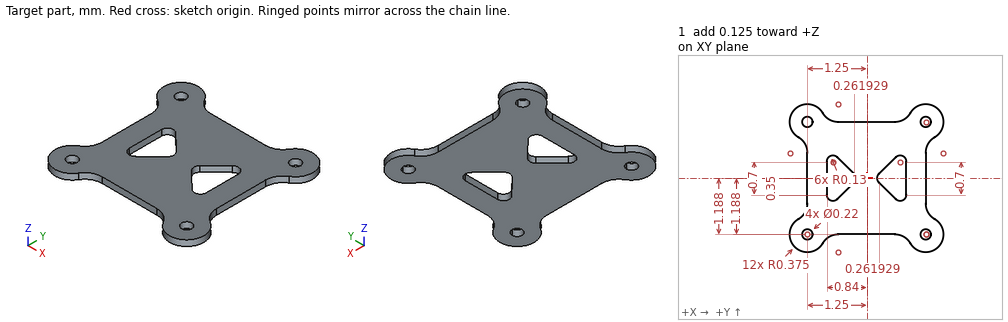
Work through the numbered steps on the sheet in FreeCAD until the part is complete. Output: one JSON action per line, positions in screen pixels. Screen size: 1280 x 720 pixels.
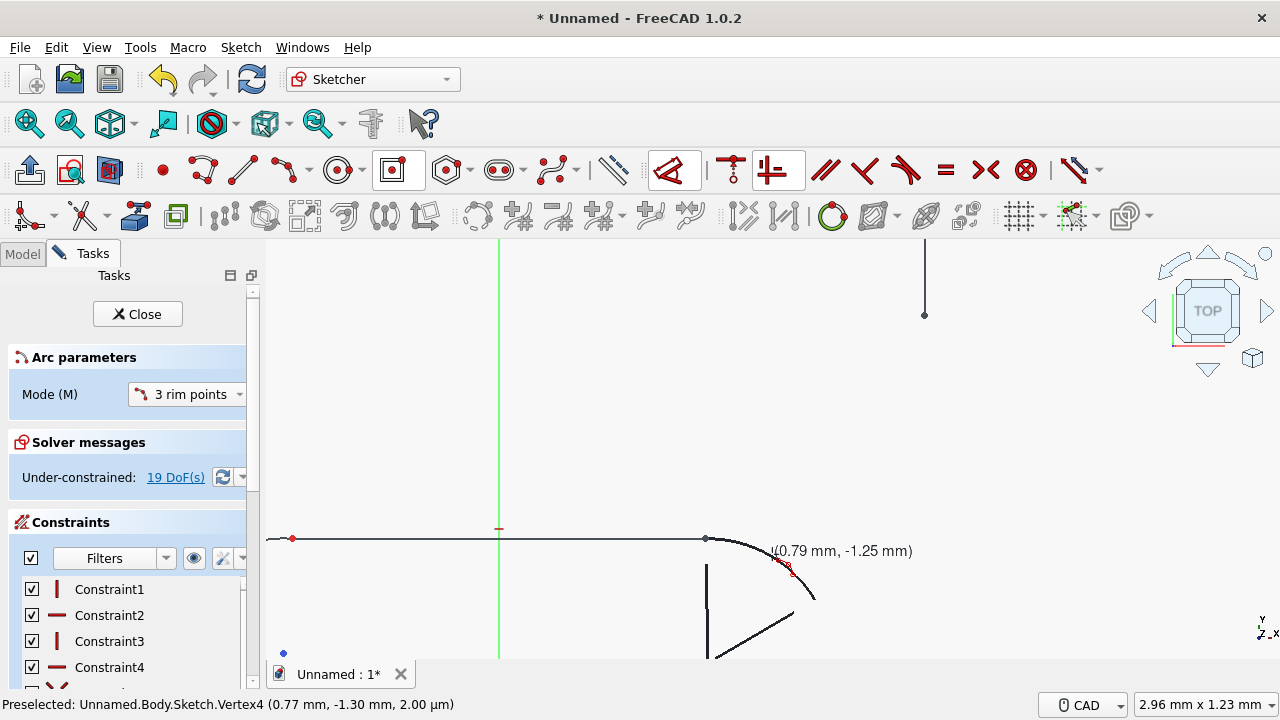
{"action": "left_click", "coordinate": [769, 551]}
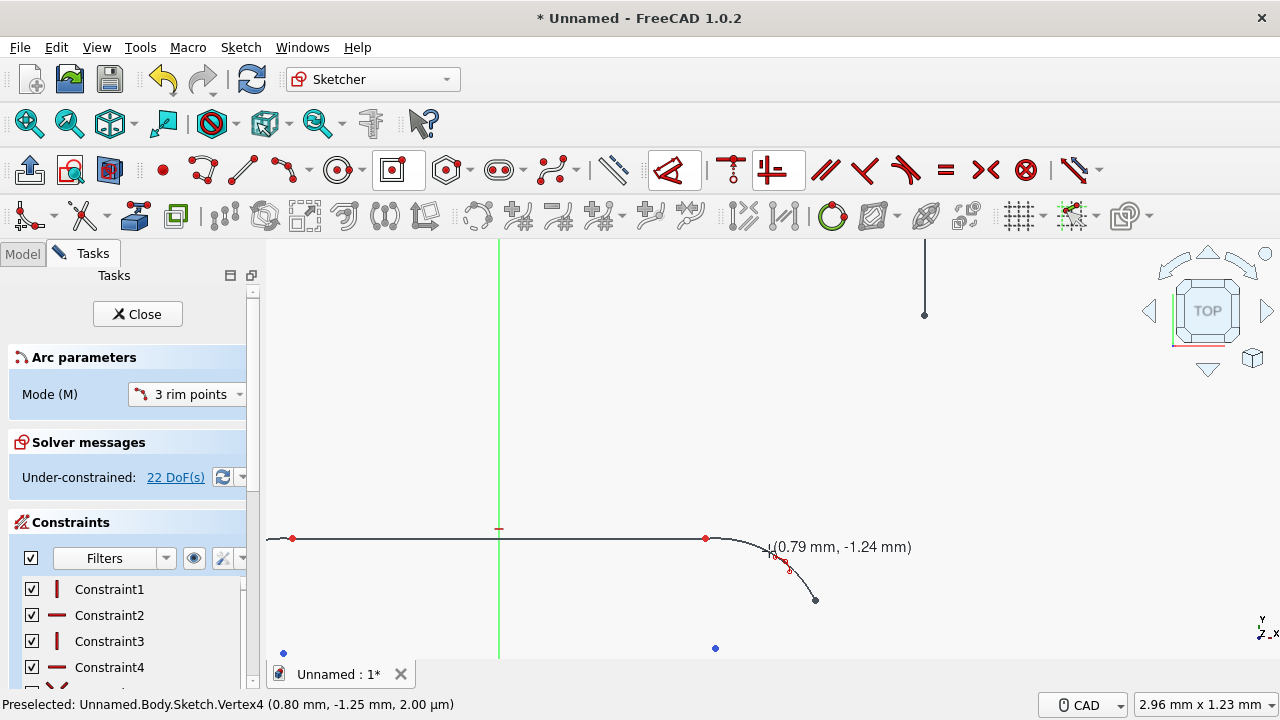
{"action": "scroll", "coordinate": [772, 554], "scroll_direction": "down", "scroll_amount": 7}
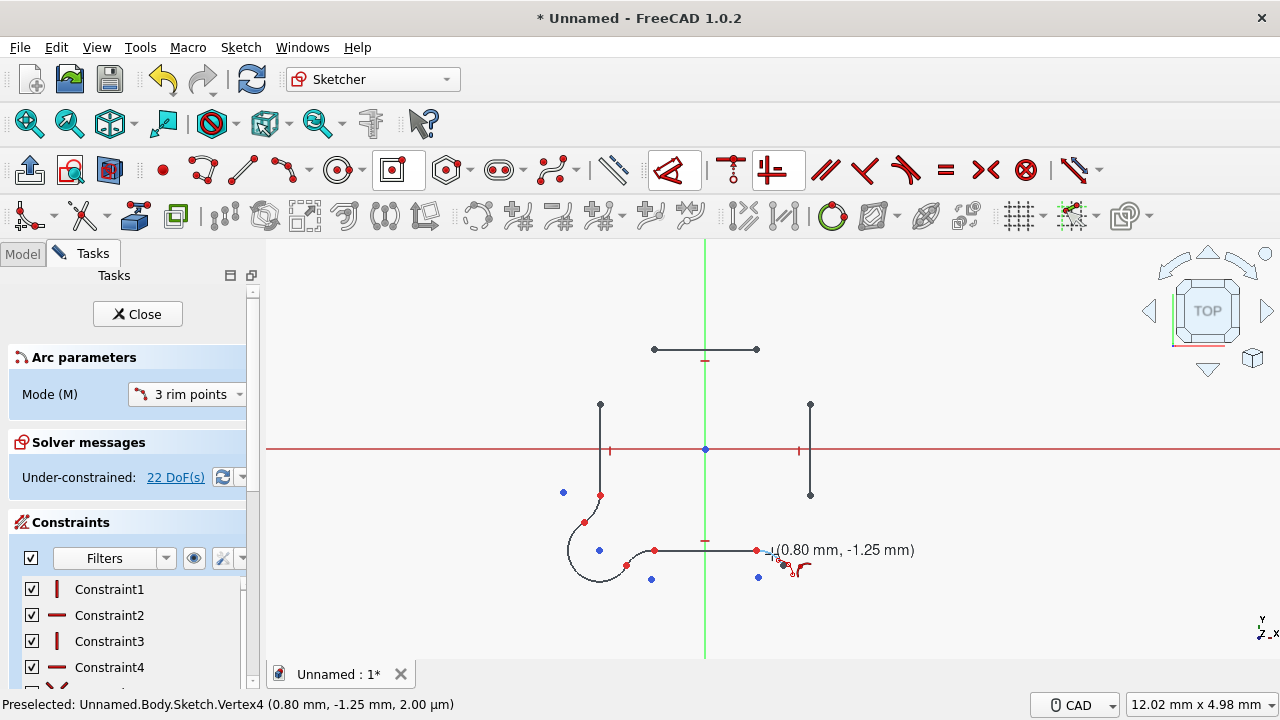
{"action": "left_click", "coordinate": [783, 566]}
{"action": "left_click", "coordinate": [826, 522]}
{"action": "left_click", "coordinate": [833, 572]}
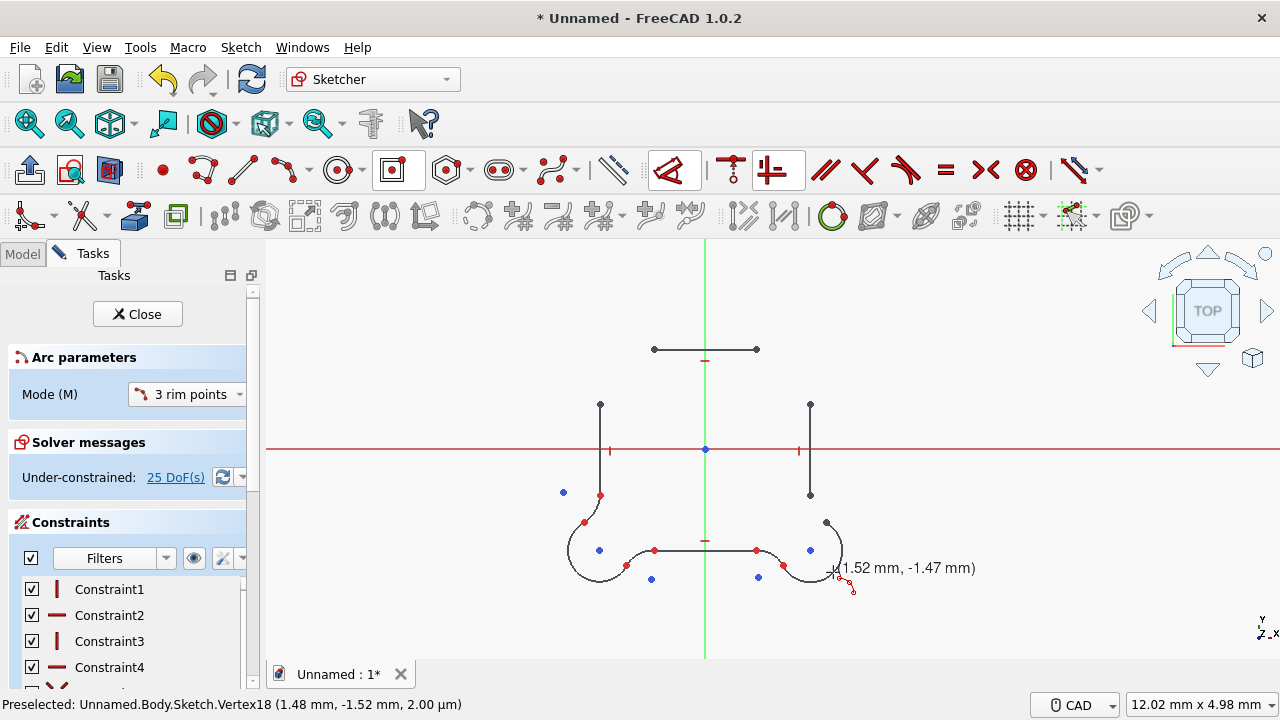
{"action": "left_click", "coordinate": [826, 523]}
{"action": "left_click", "coordinate": [810, 496]}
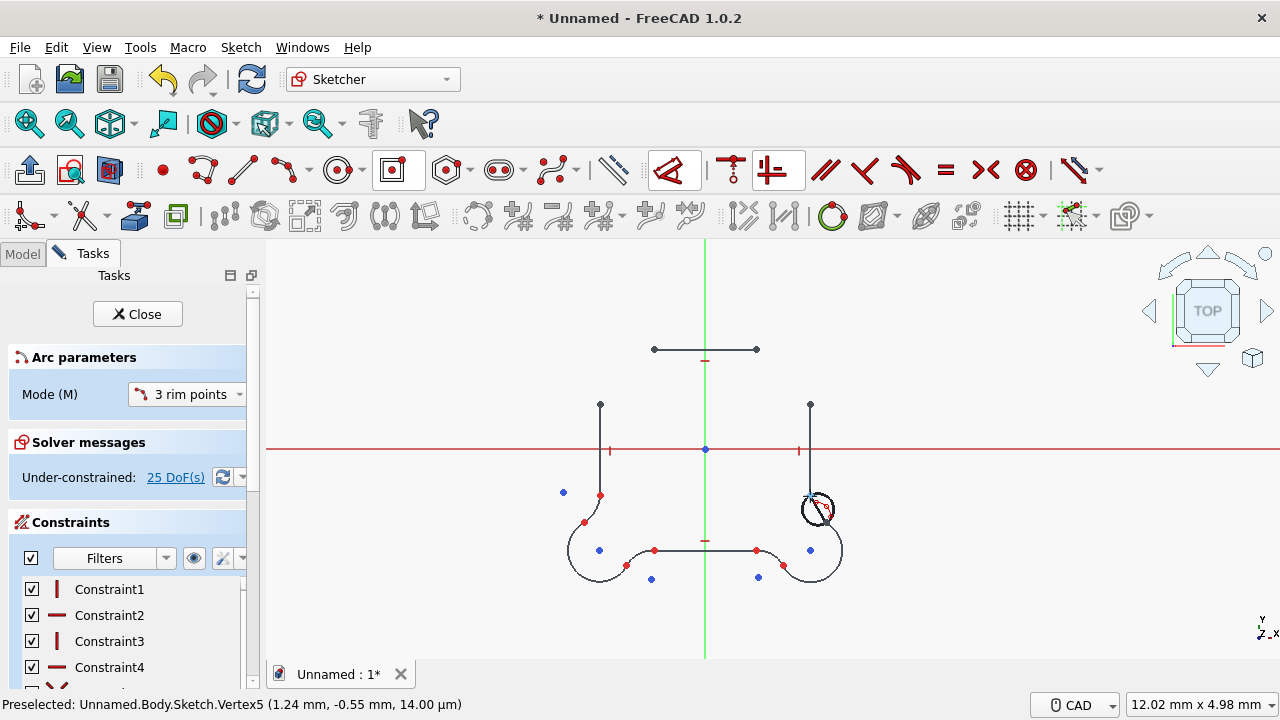
{"action": "scroll", "coordinate": [815, 510], "scroll_direction": "up", "scroll_amount": 7}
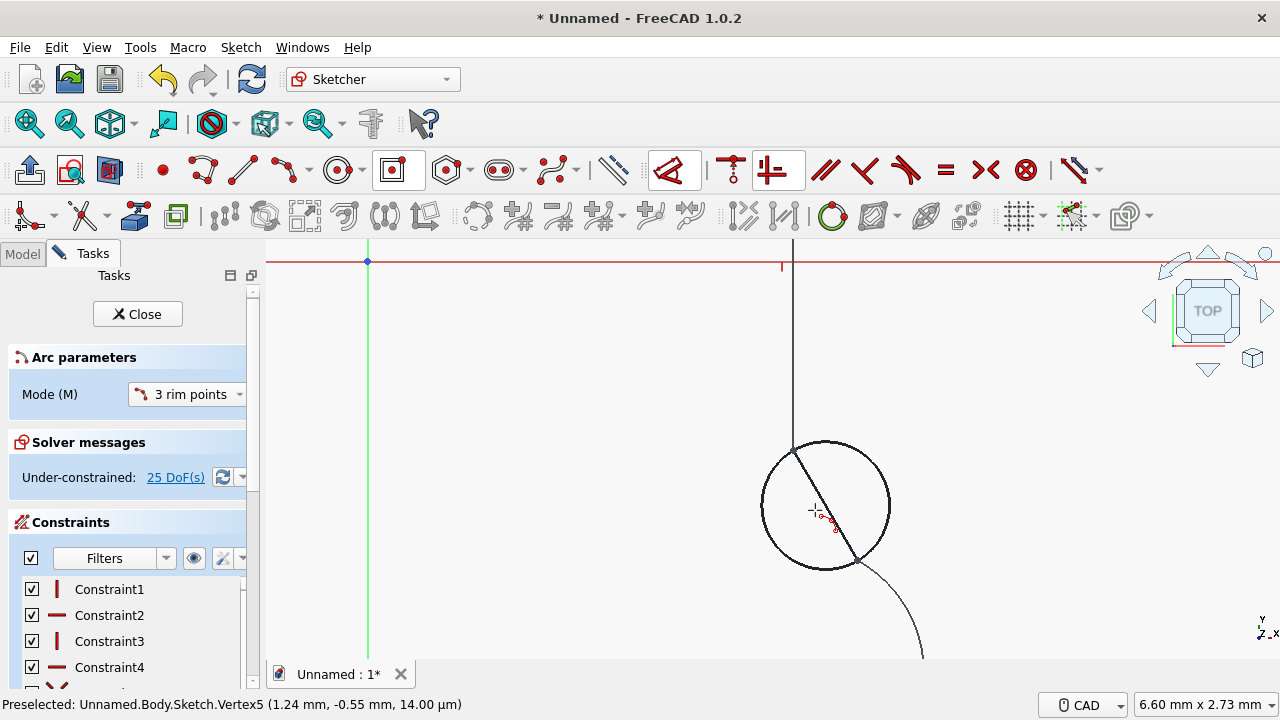
{"action": "left_click", "coordinate": [813, 510]}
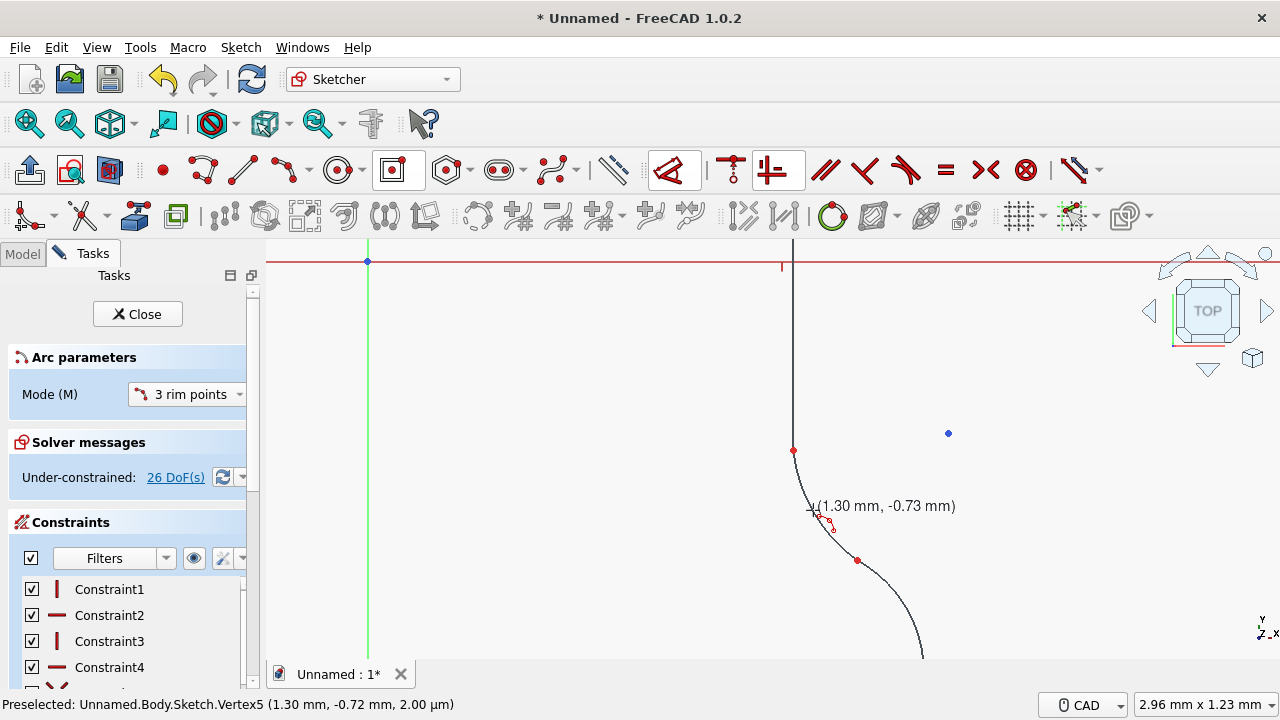
{"action": "scroll", "coordinate": [815, 510], "scroll_direction": "down", "scroll_amount": 7}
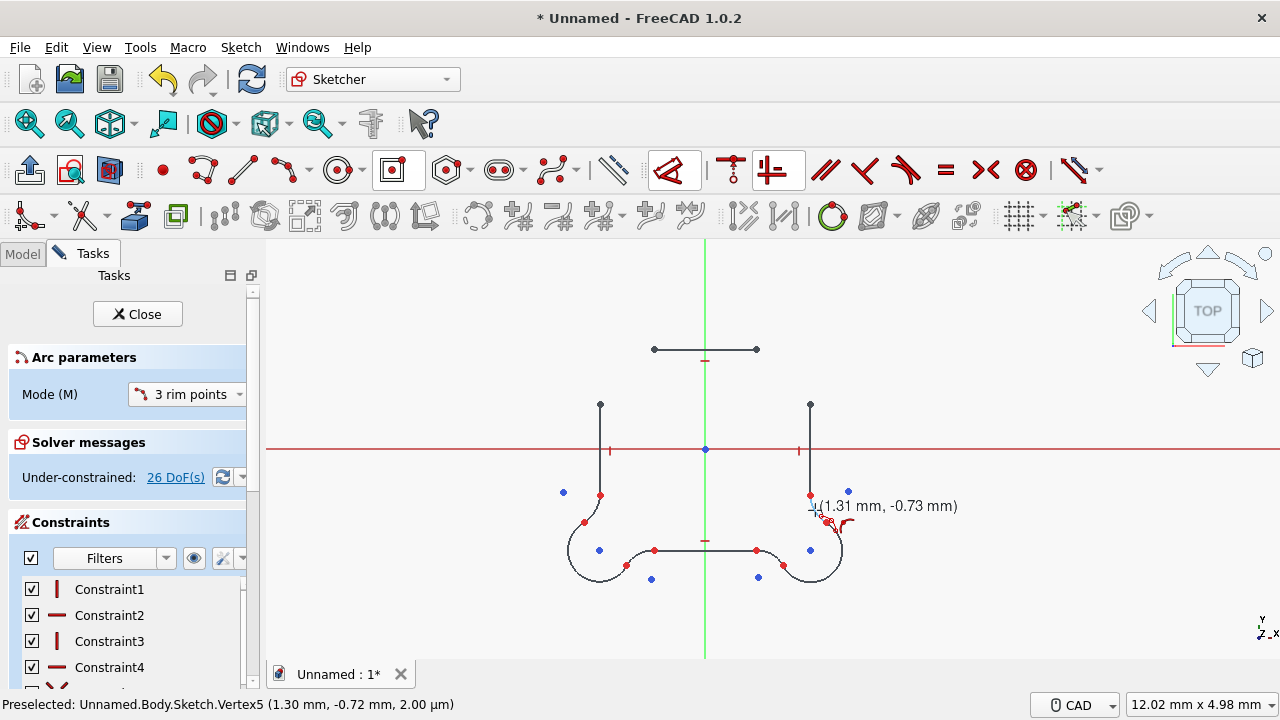
{"action": "left_click", "coordinate": [810, 405]}
{"action": "left_click", "coordinate": [826, 376]}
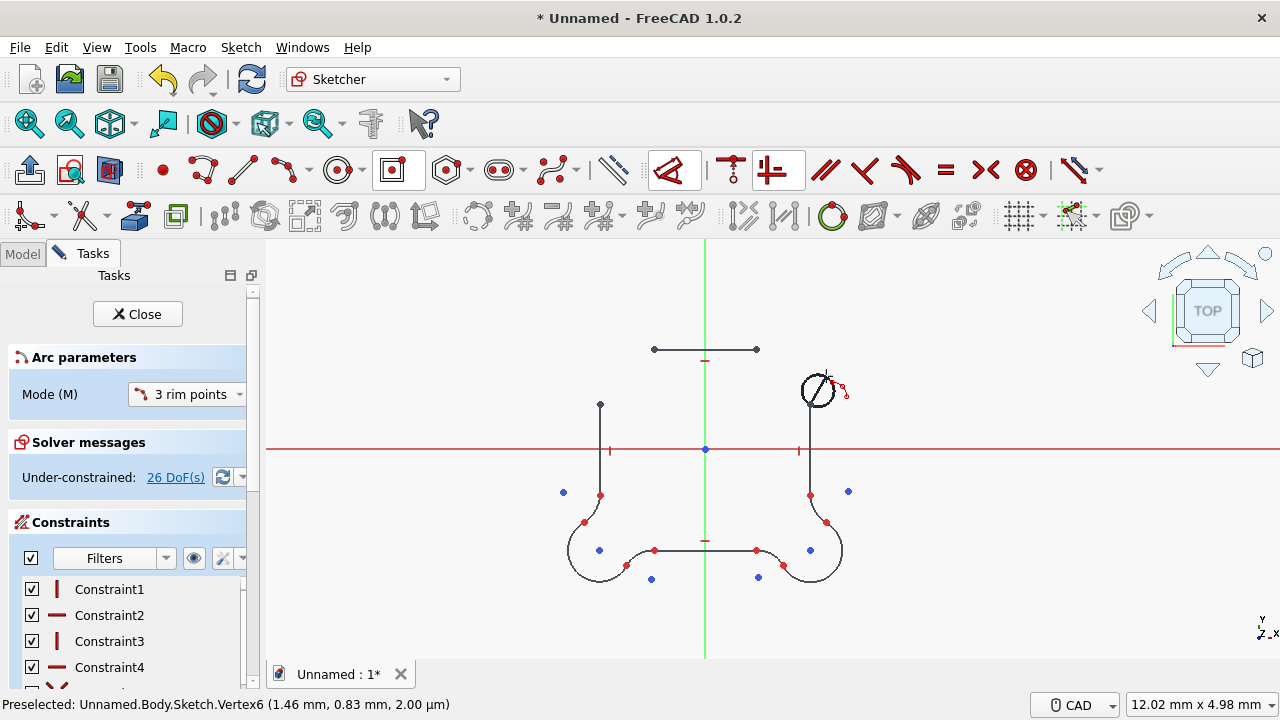
{"action": "scroll", "coordinate": [815, 388], "scroll_direction": "up", "scroll_amount": 7}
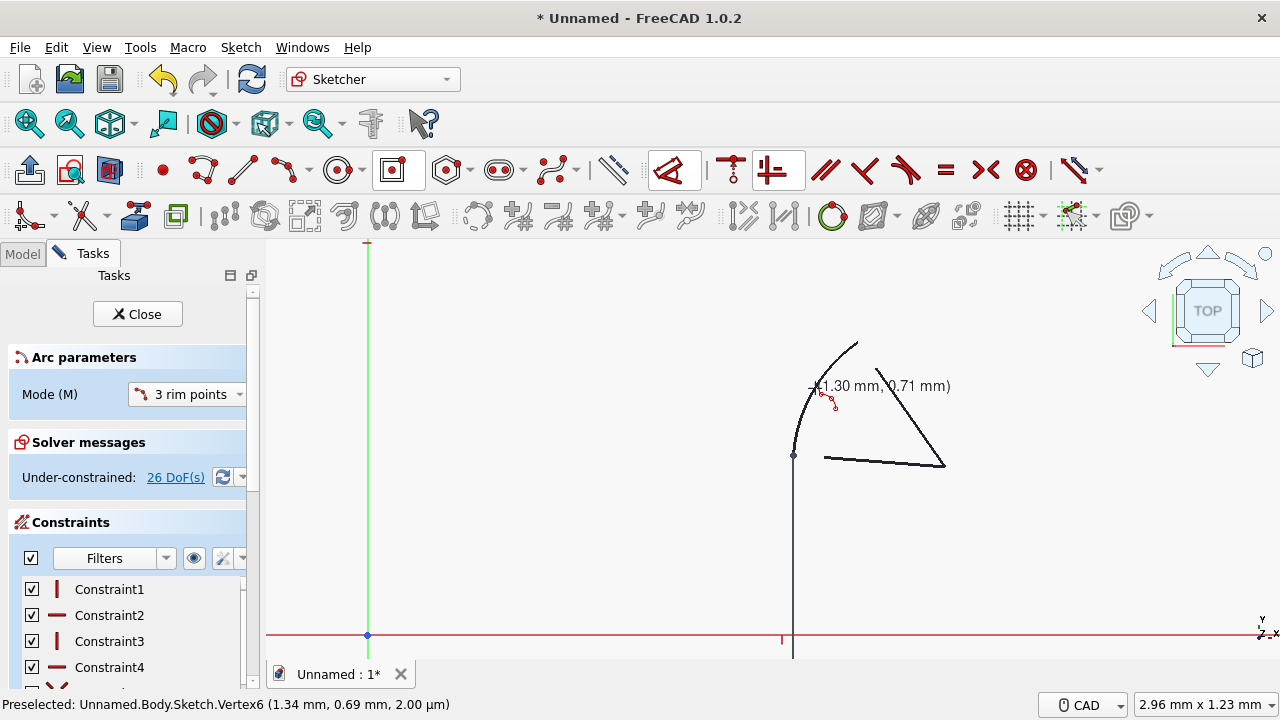
{"action": "left_click", "coordinate": [813, 387]}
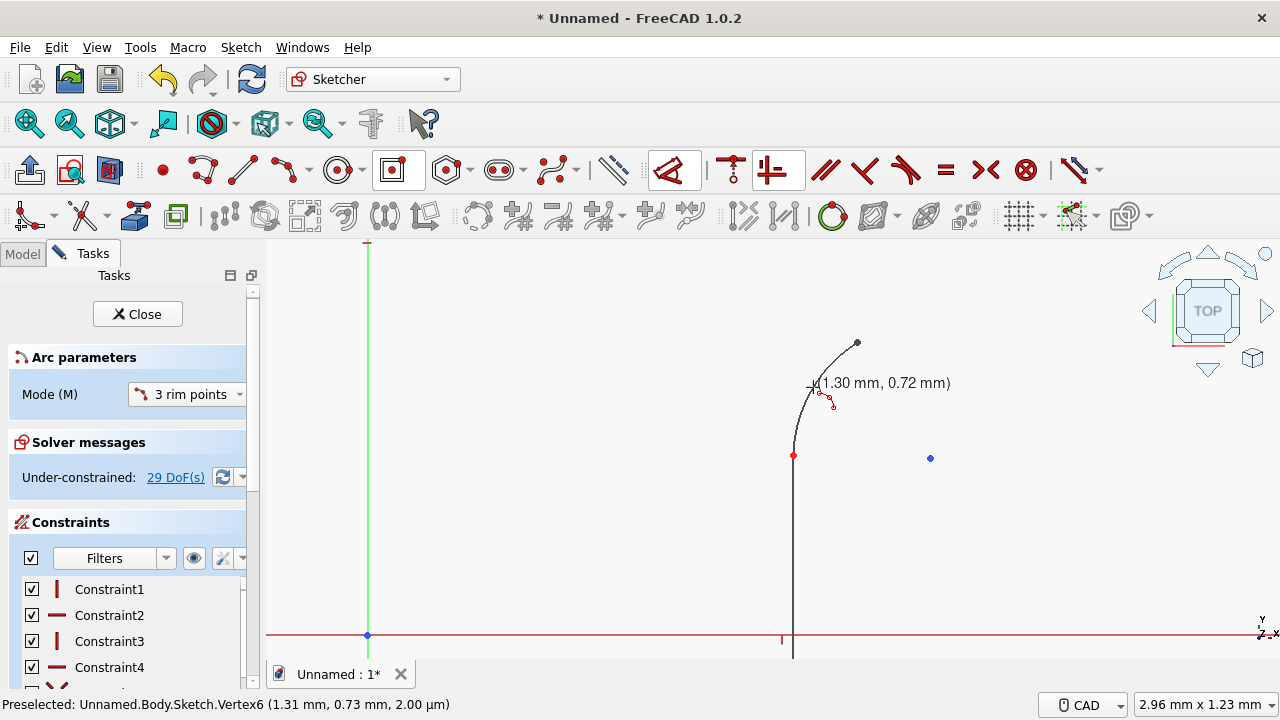
{"action": "scroll", "coordinate": [815, 388], "scroll_direction": "down", "scroll_amount": 7}